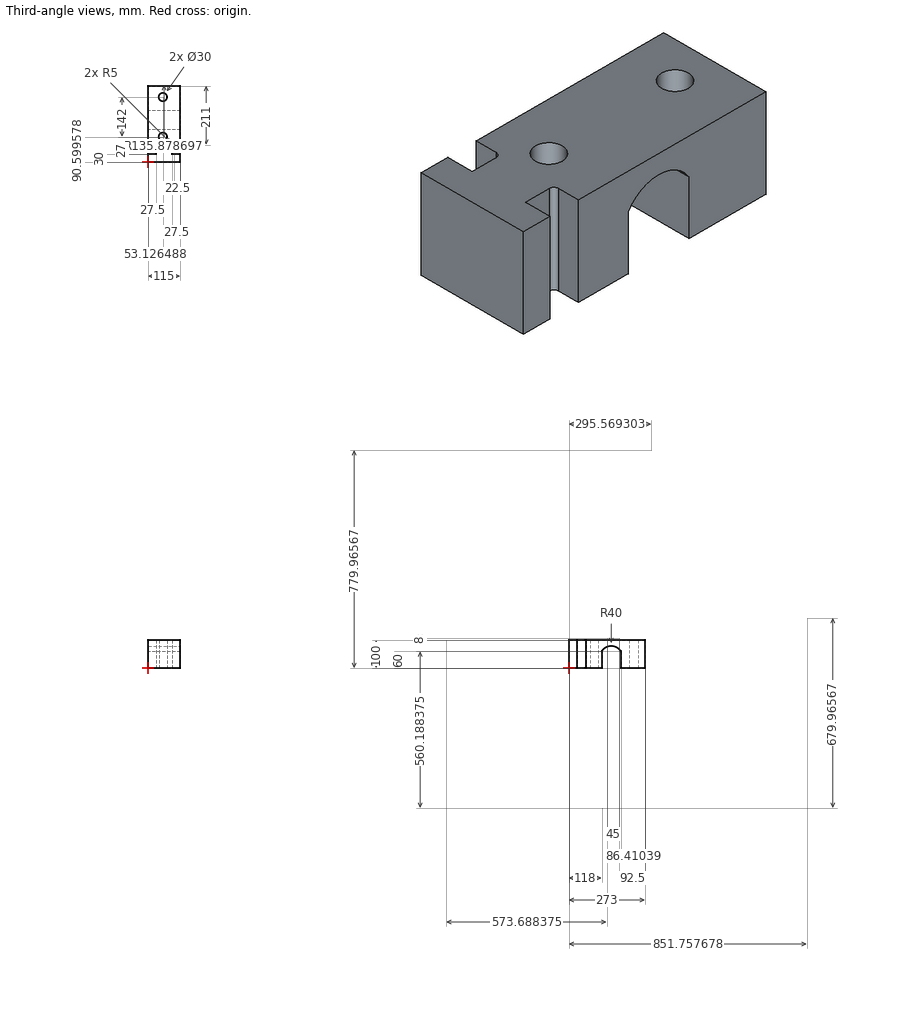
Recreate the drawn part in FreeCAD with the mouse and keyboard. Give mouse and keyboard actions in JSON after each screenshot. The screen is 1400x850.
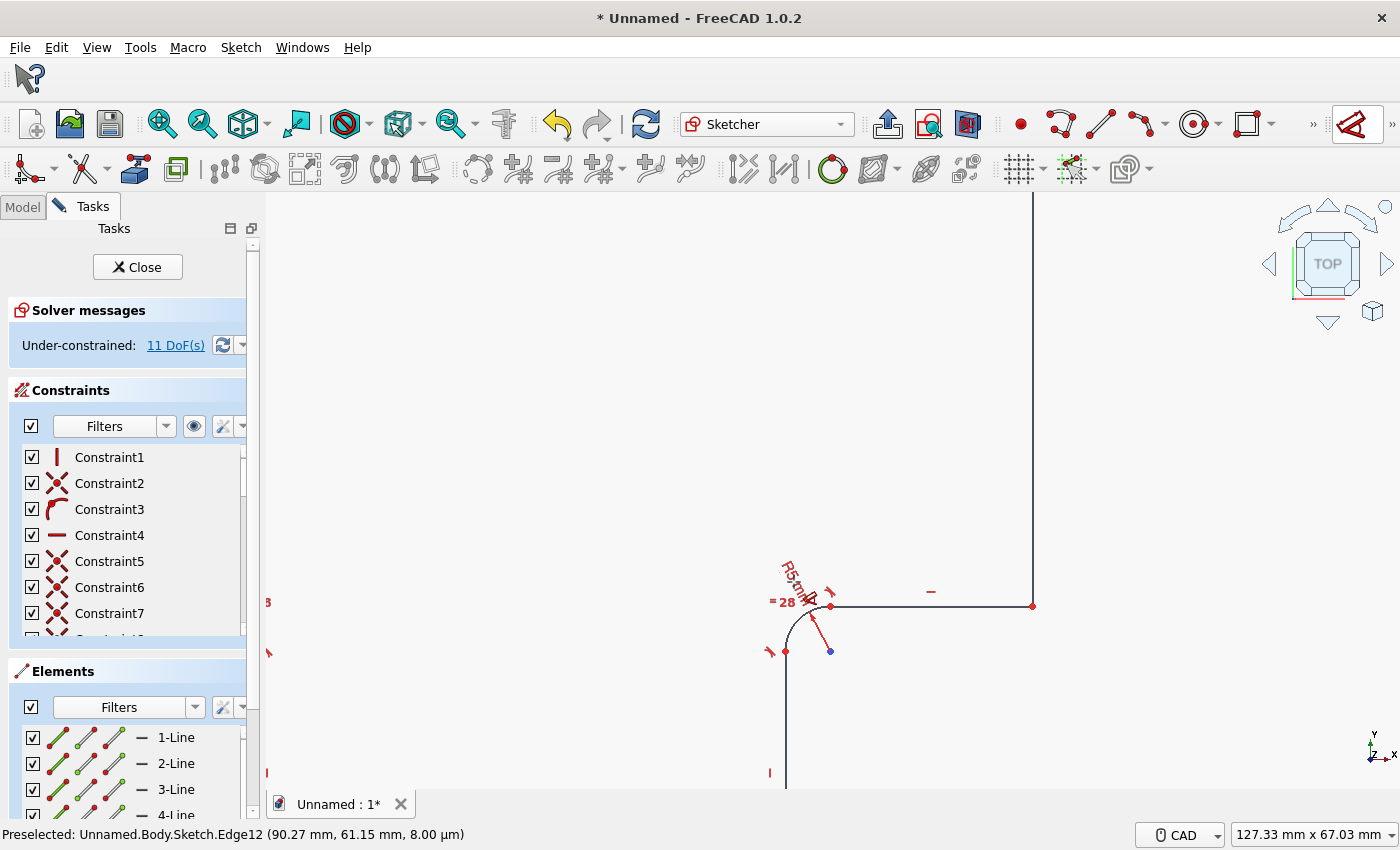
{"action": "scroll", "coordinate": [813, 611], "scroll_direction": "down", "scroll_amount": 9}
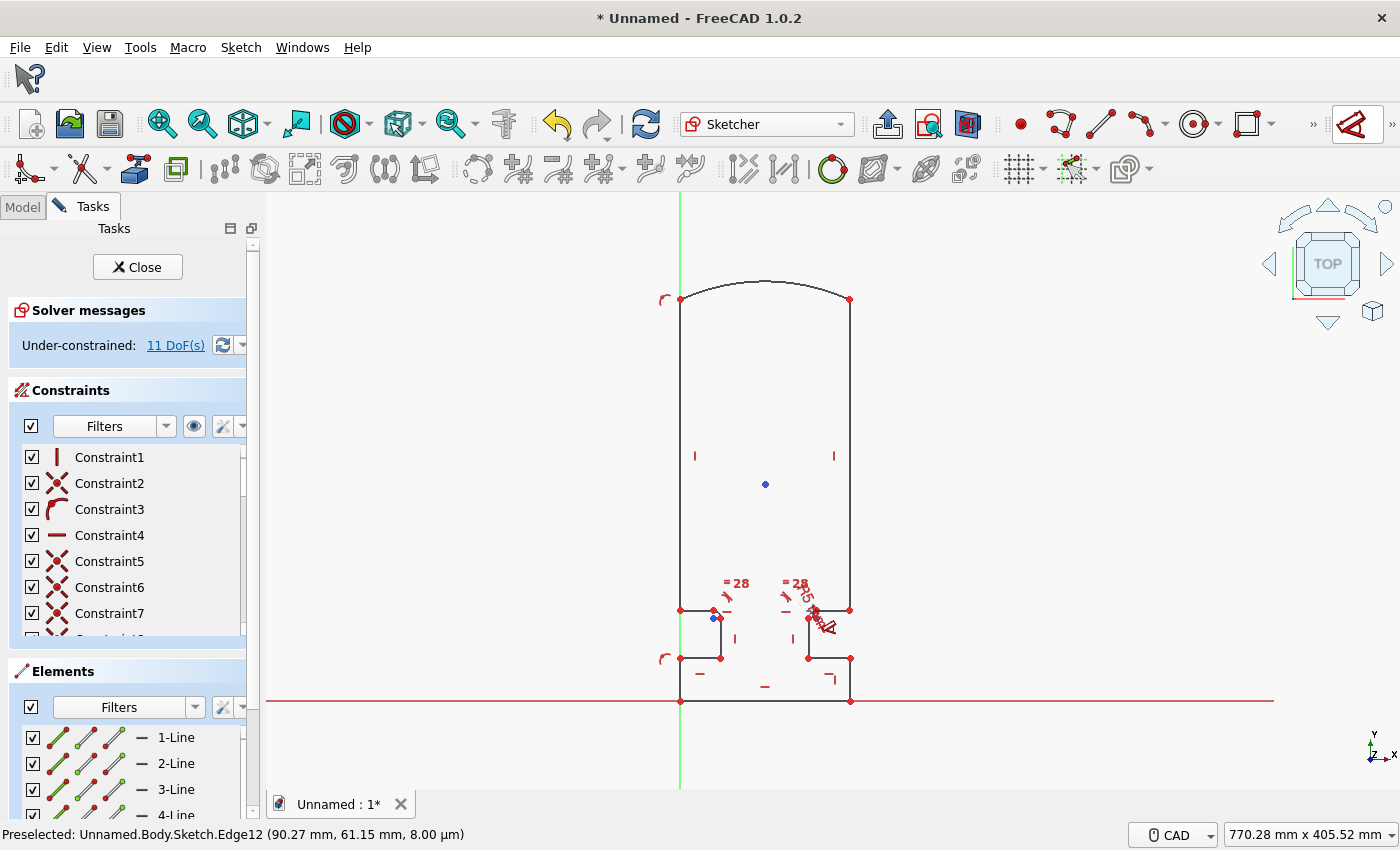
{"action": "left_click", "coordinate": [800, 284]}
{"action": "left_click", "coordinate": [805, 252]}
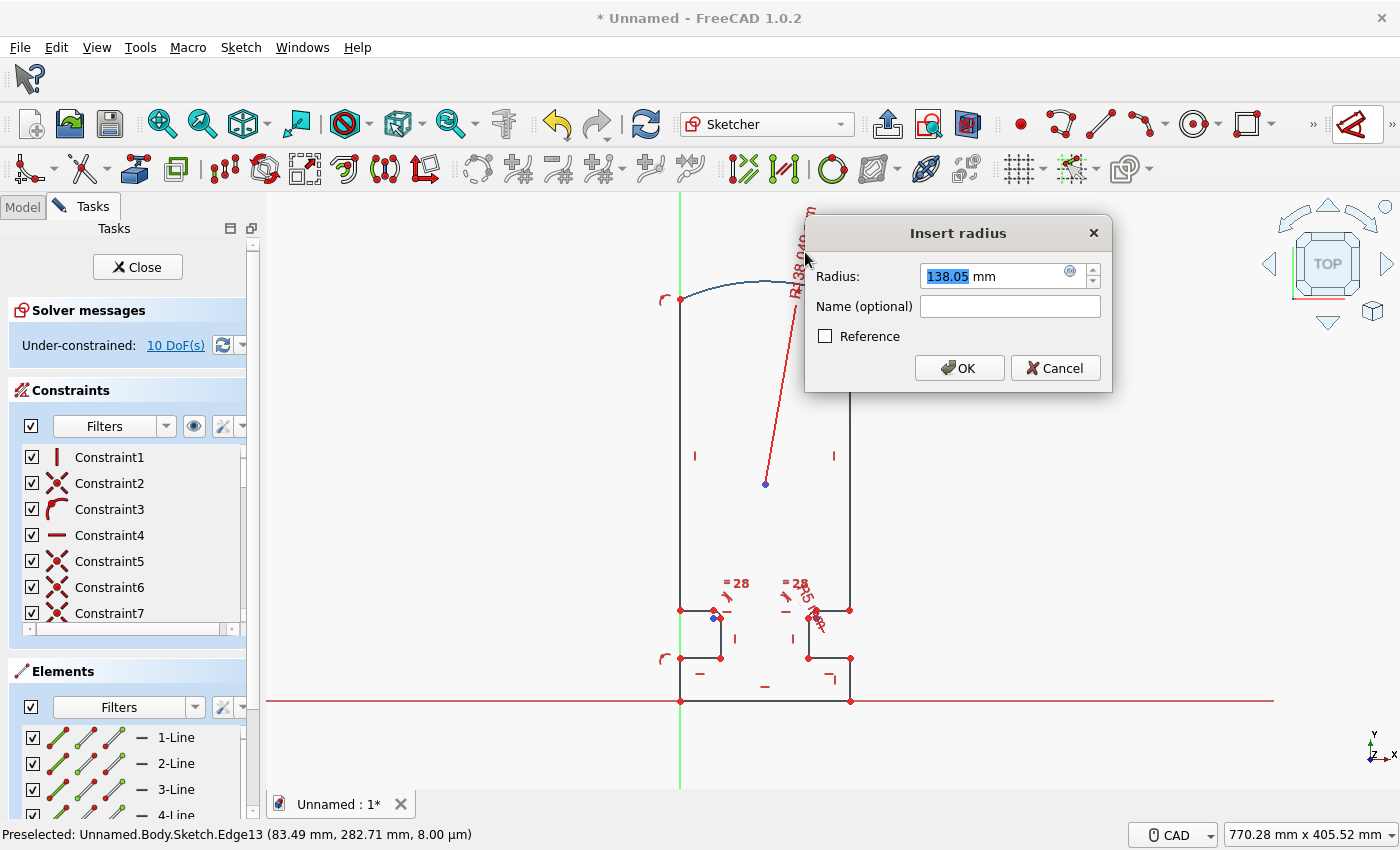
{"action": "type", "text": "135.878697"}
{"action": "key", "text": "Return"}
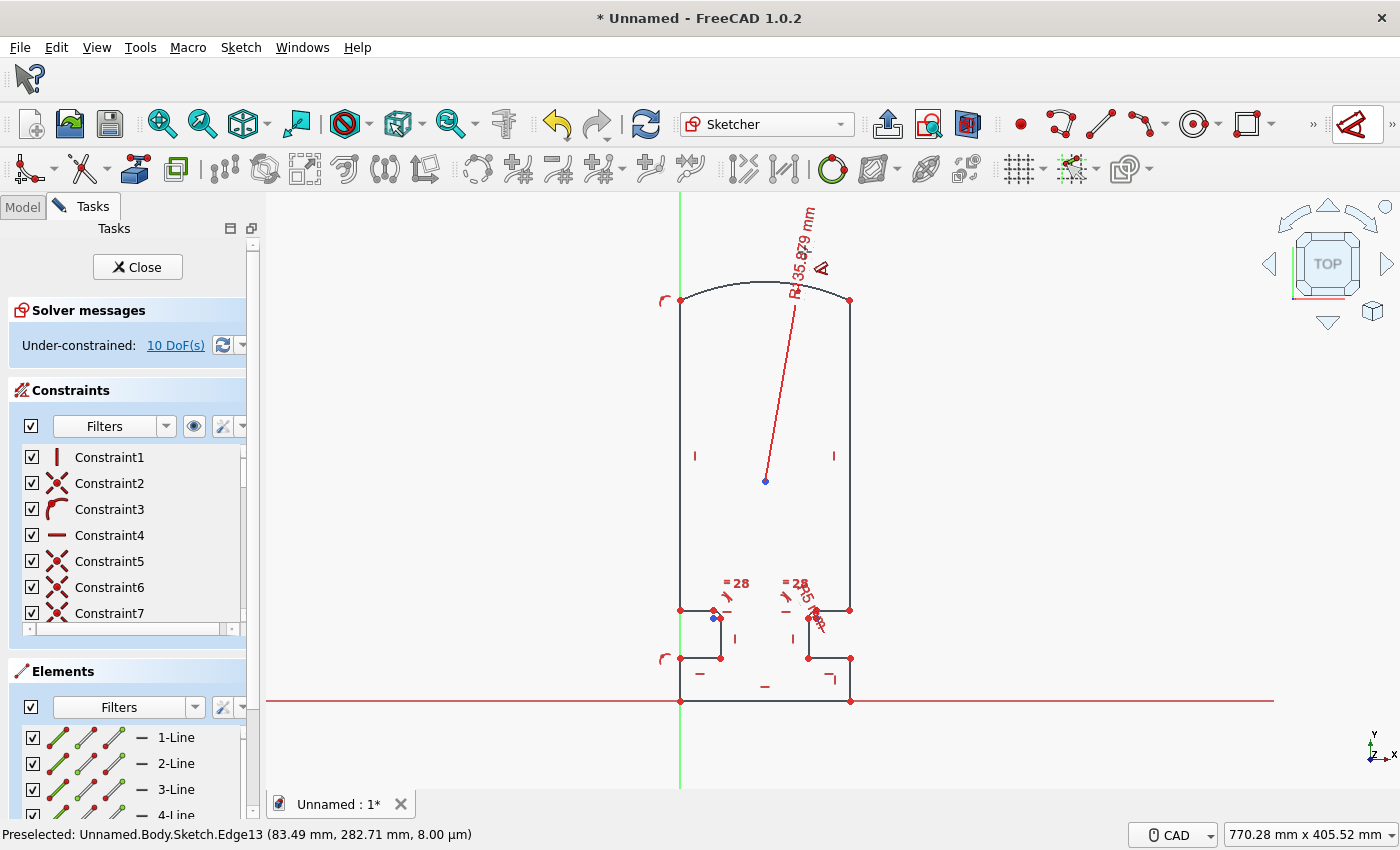
{"action": "left_click", "coordinate": [721, 630]}
{"action": "left_click", "coordinate": [755, 638]}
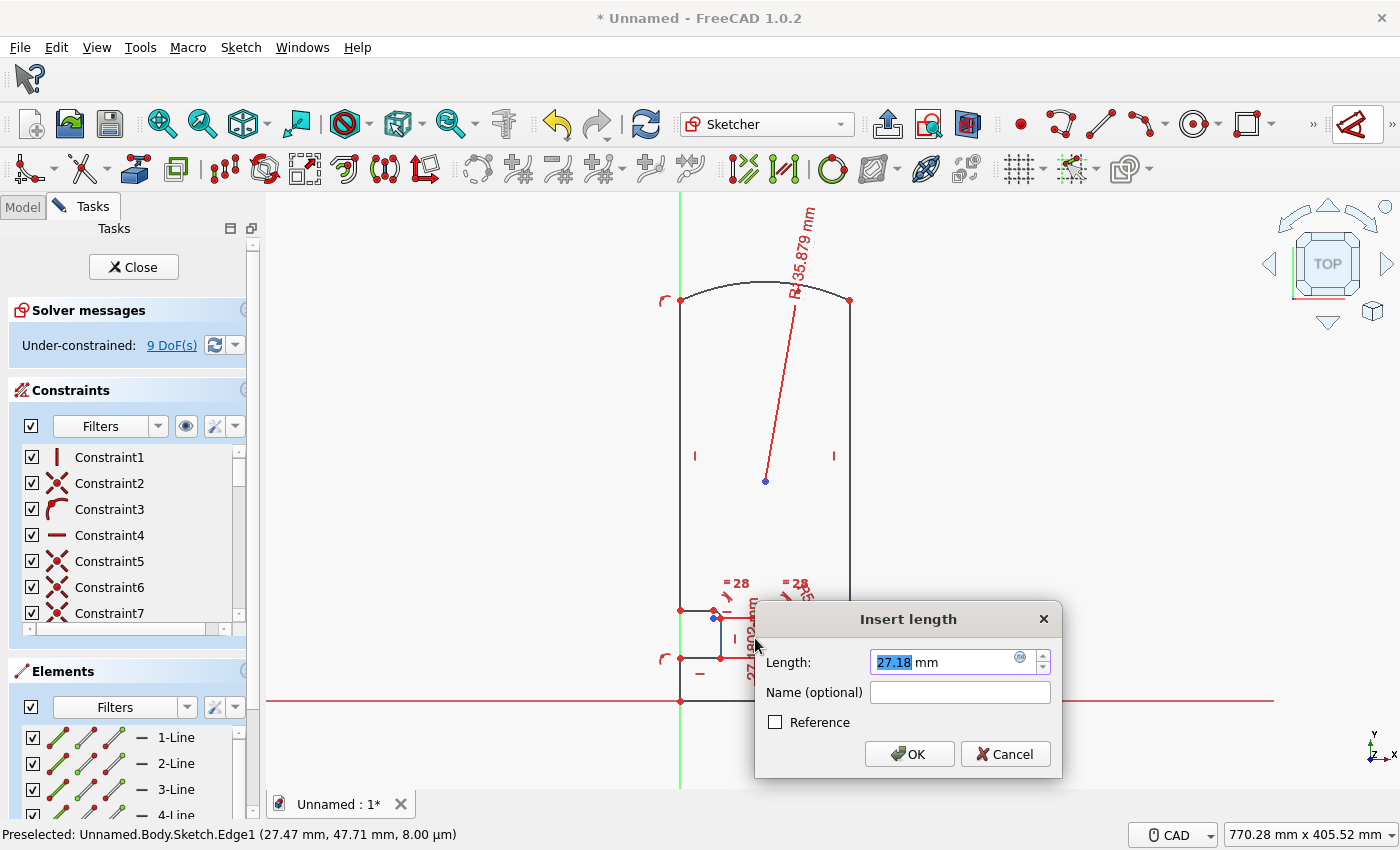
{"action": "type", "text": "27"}
{"action": "key", "text": "Return"}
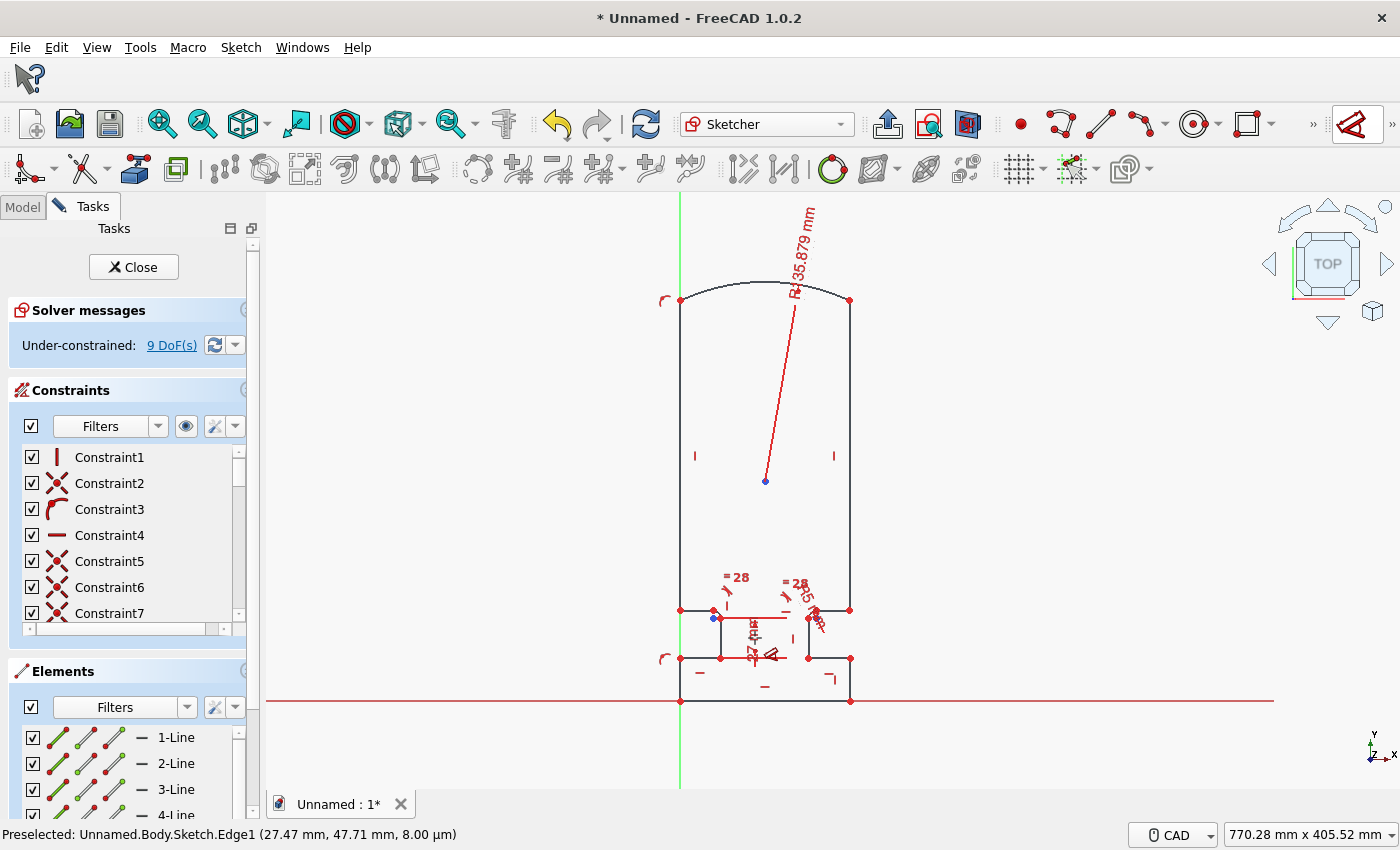
{"action": "left_click", "coordinate": [680, 671]}
{"action": "left_click", "coordinate": [646, 680]}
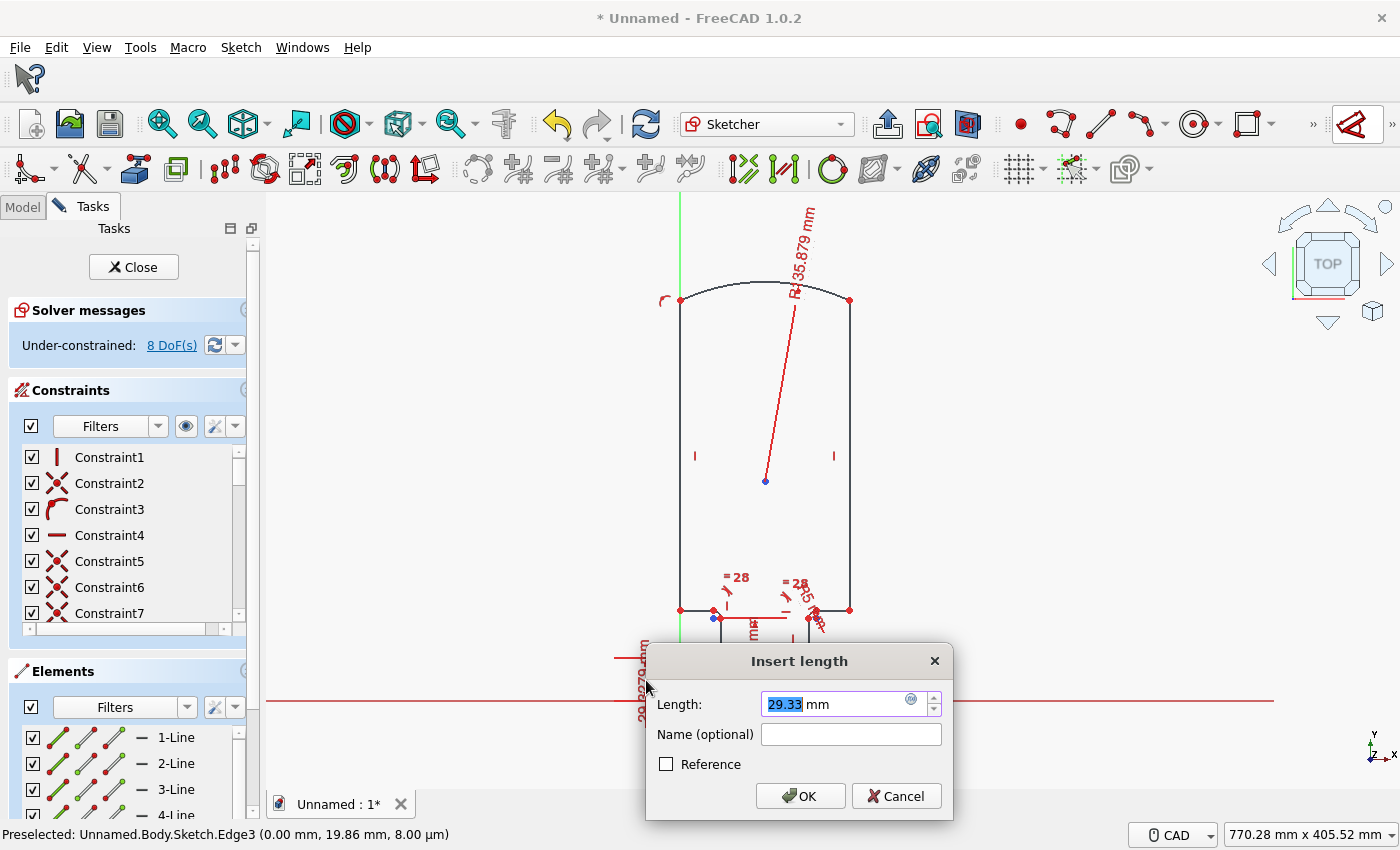
{"action": "type", "text": "30"}
{"action": "key", "text": "Return"}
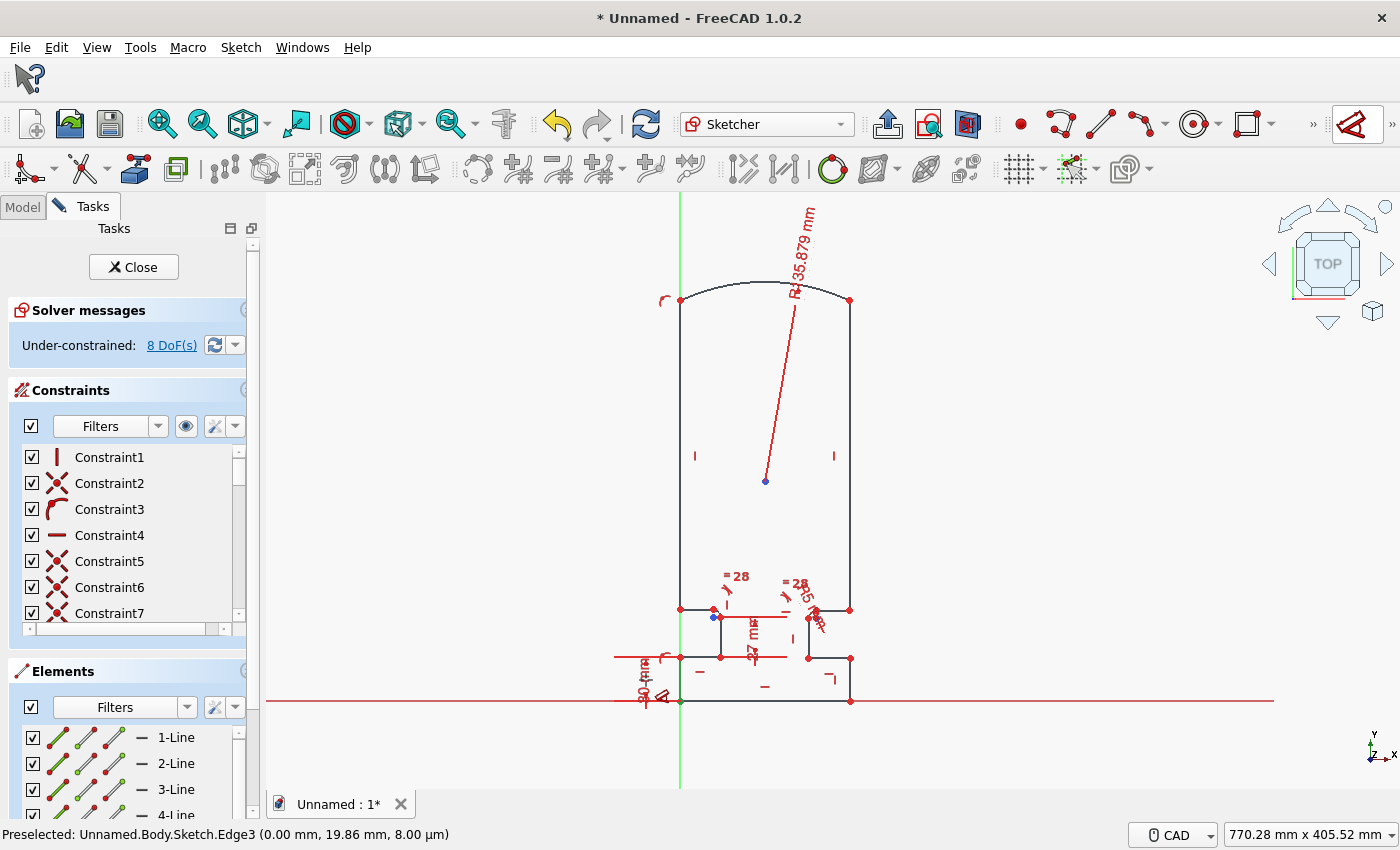
{"action": "left_click", "coordinate": [850, 688]}
{"action": "left_click", "coordinate": [884, 680]}